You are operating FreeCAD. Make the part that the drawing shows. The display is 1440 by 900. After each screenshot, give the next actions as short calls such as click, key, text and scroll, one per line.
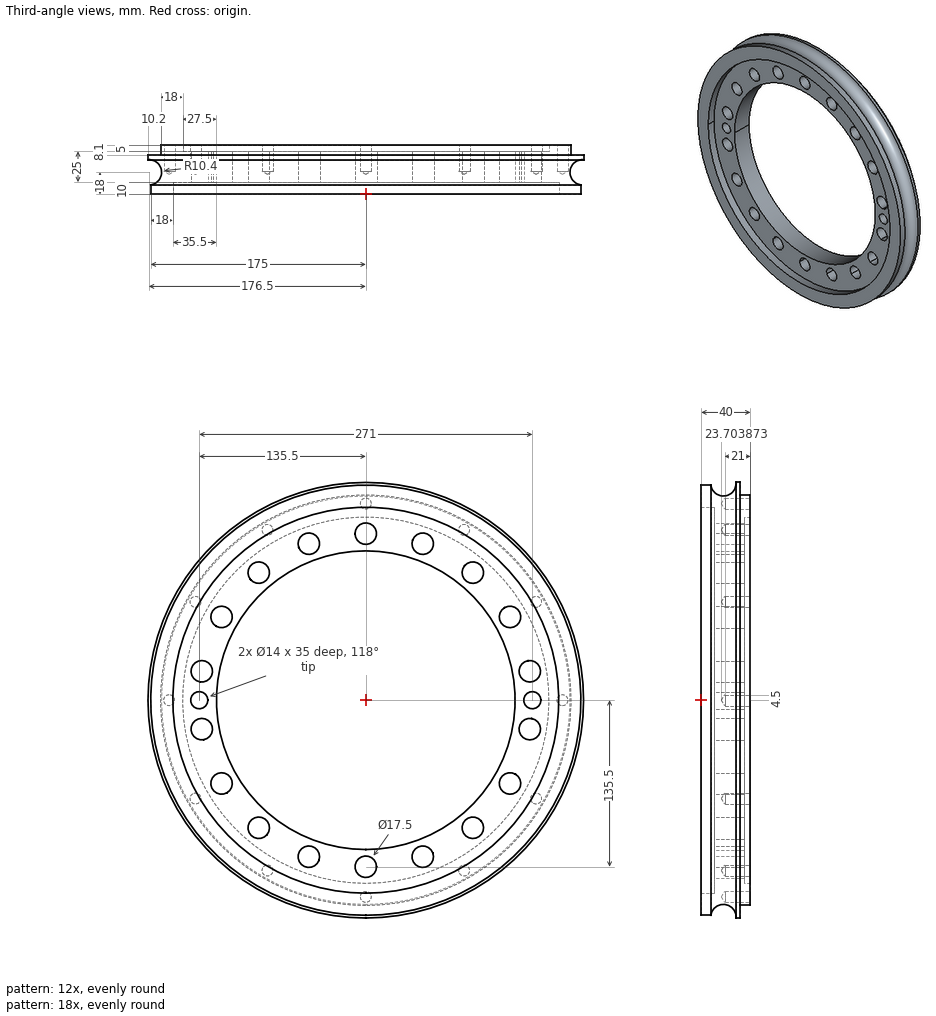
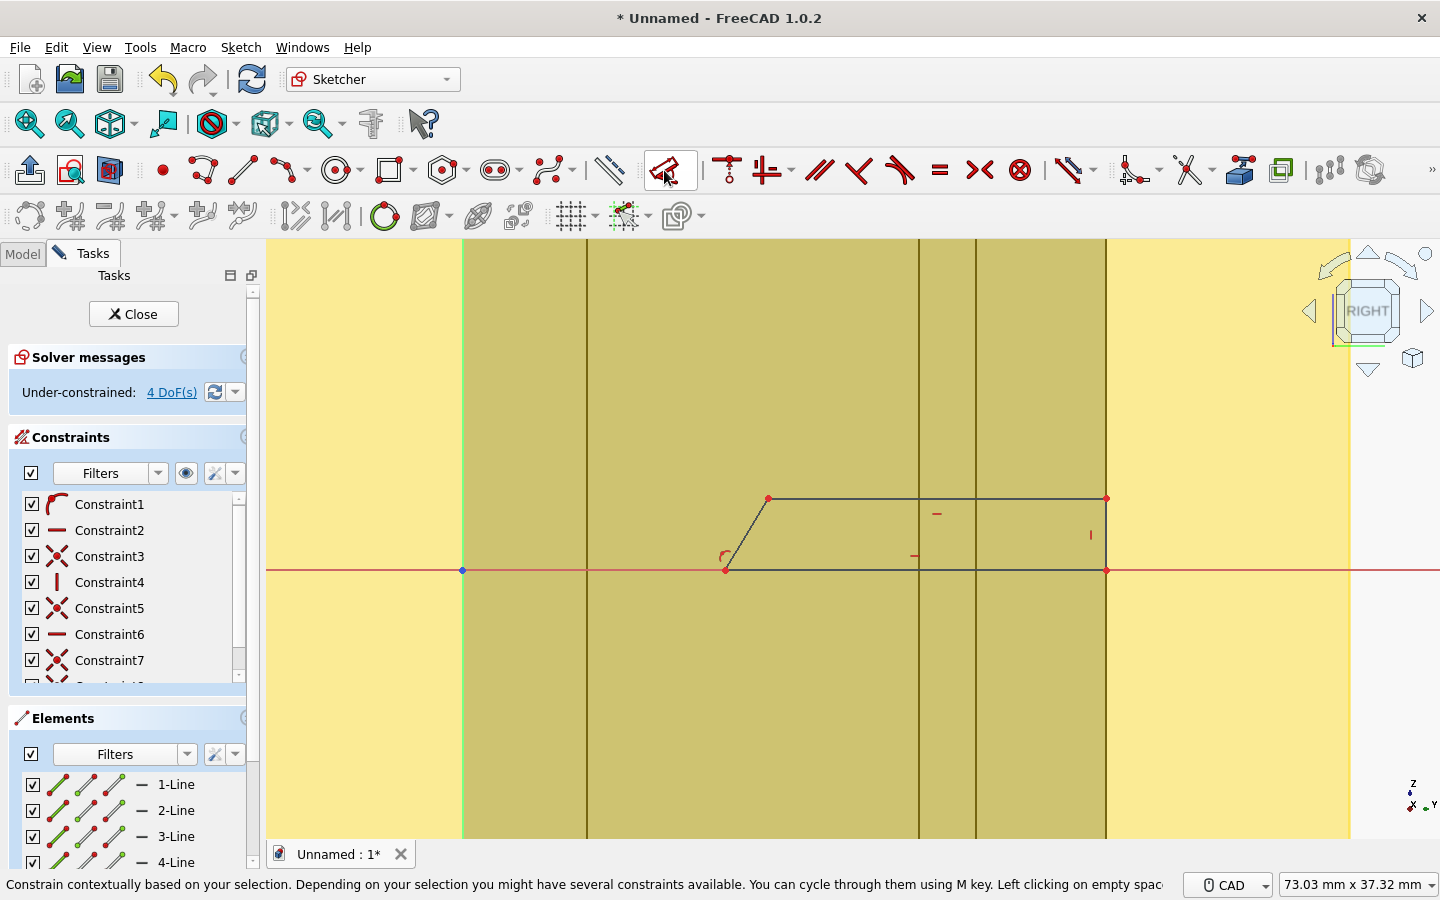
click(1005, 499)
click(937, 465)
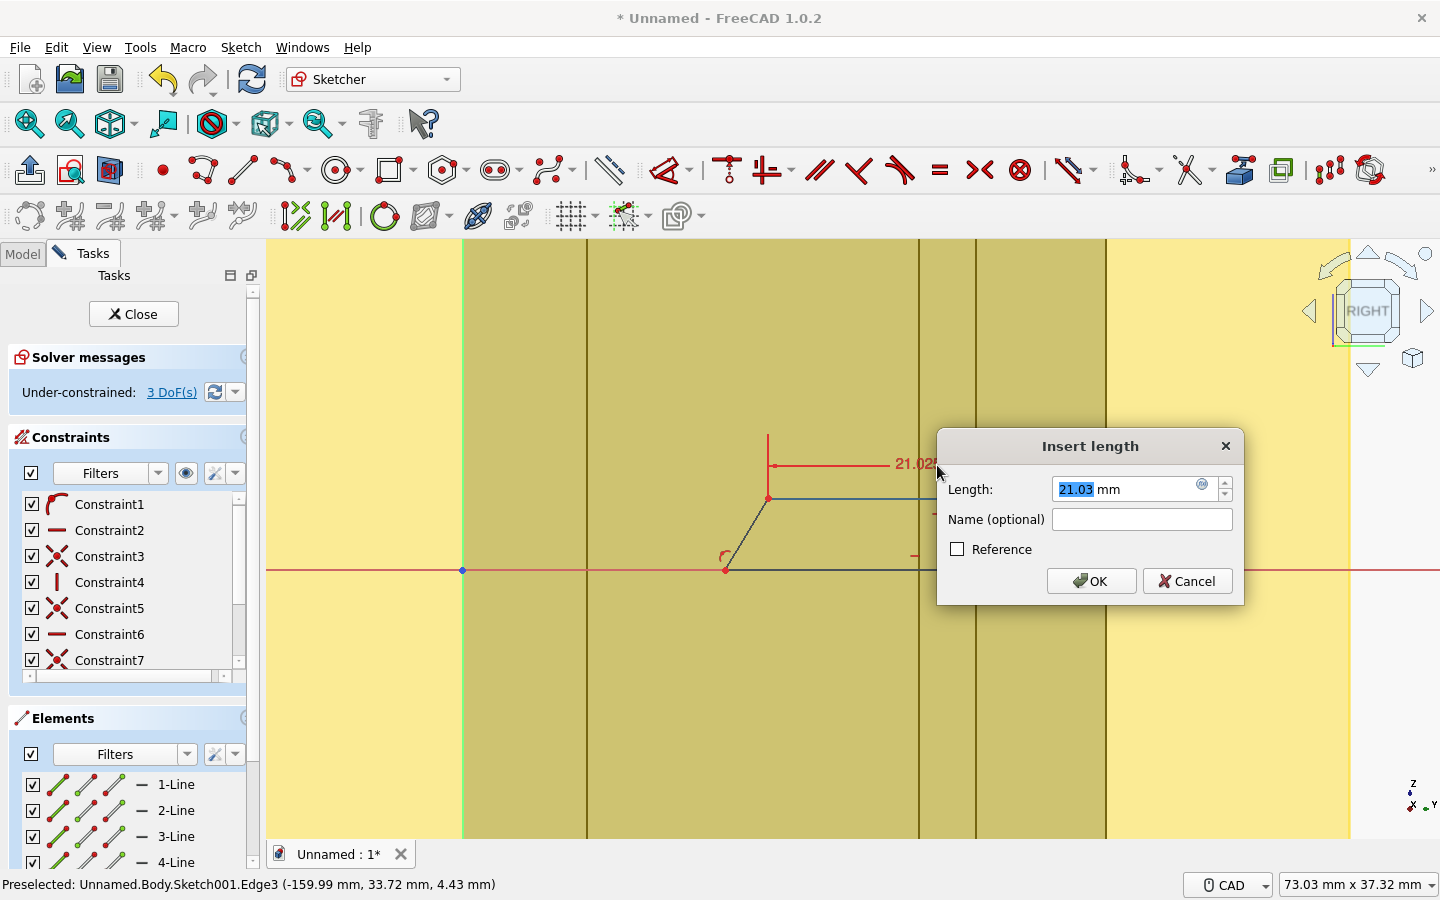
text(21)
key(Return)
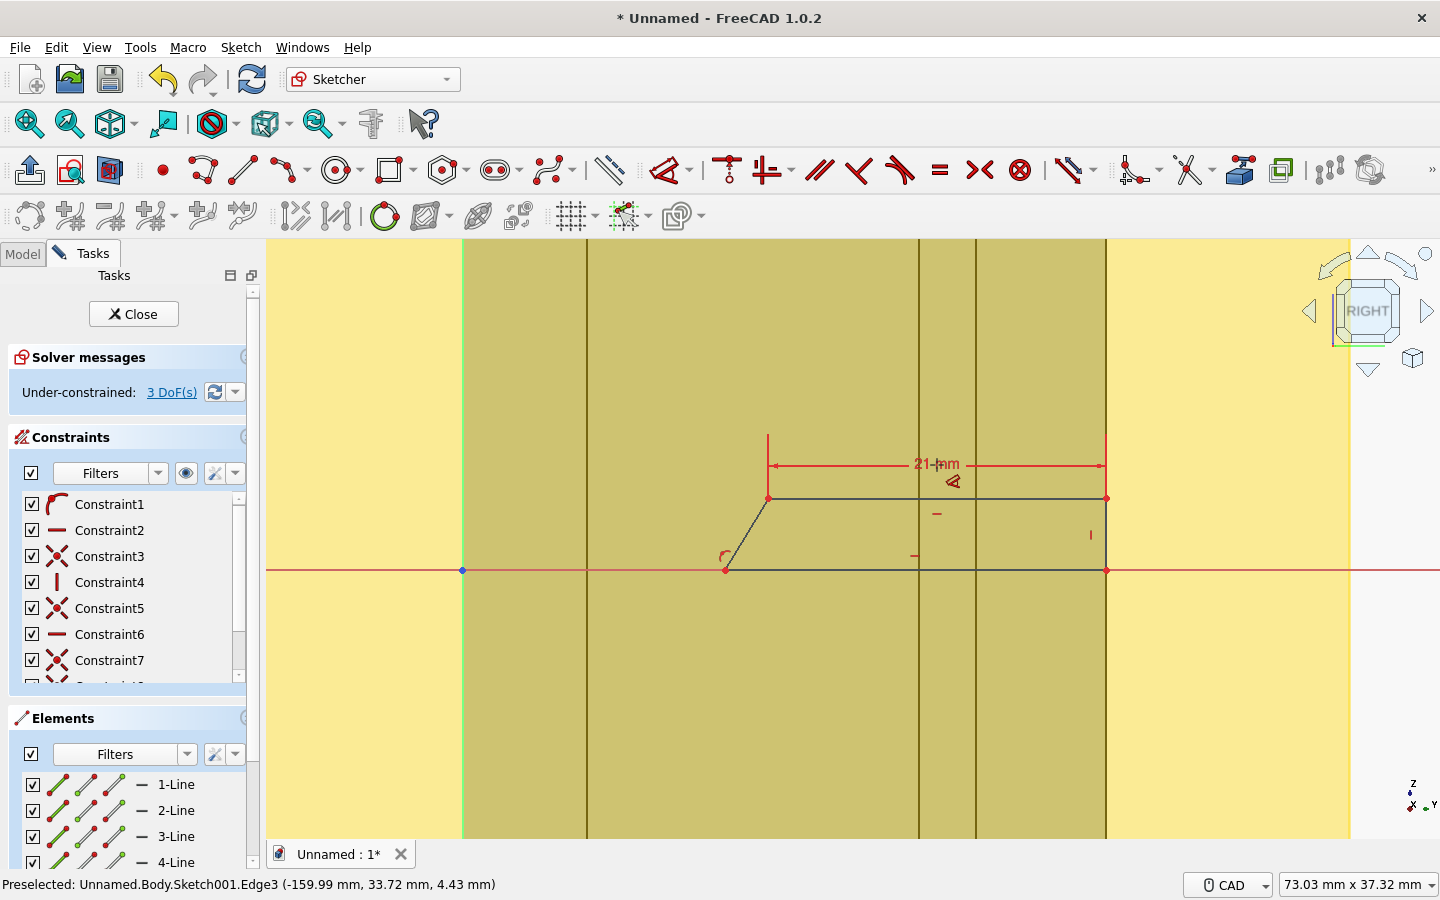
click(1106, 549)
click(1140, 535)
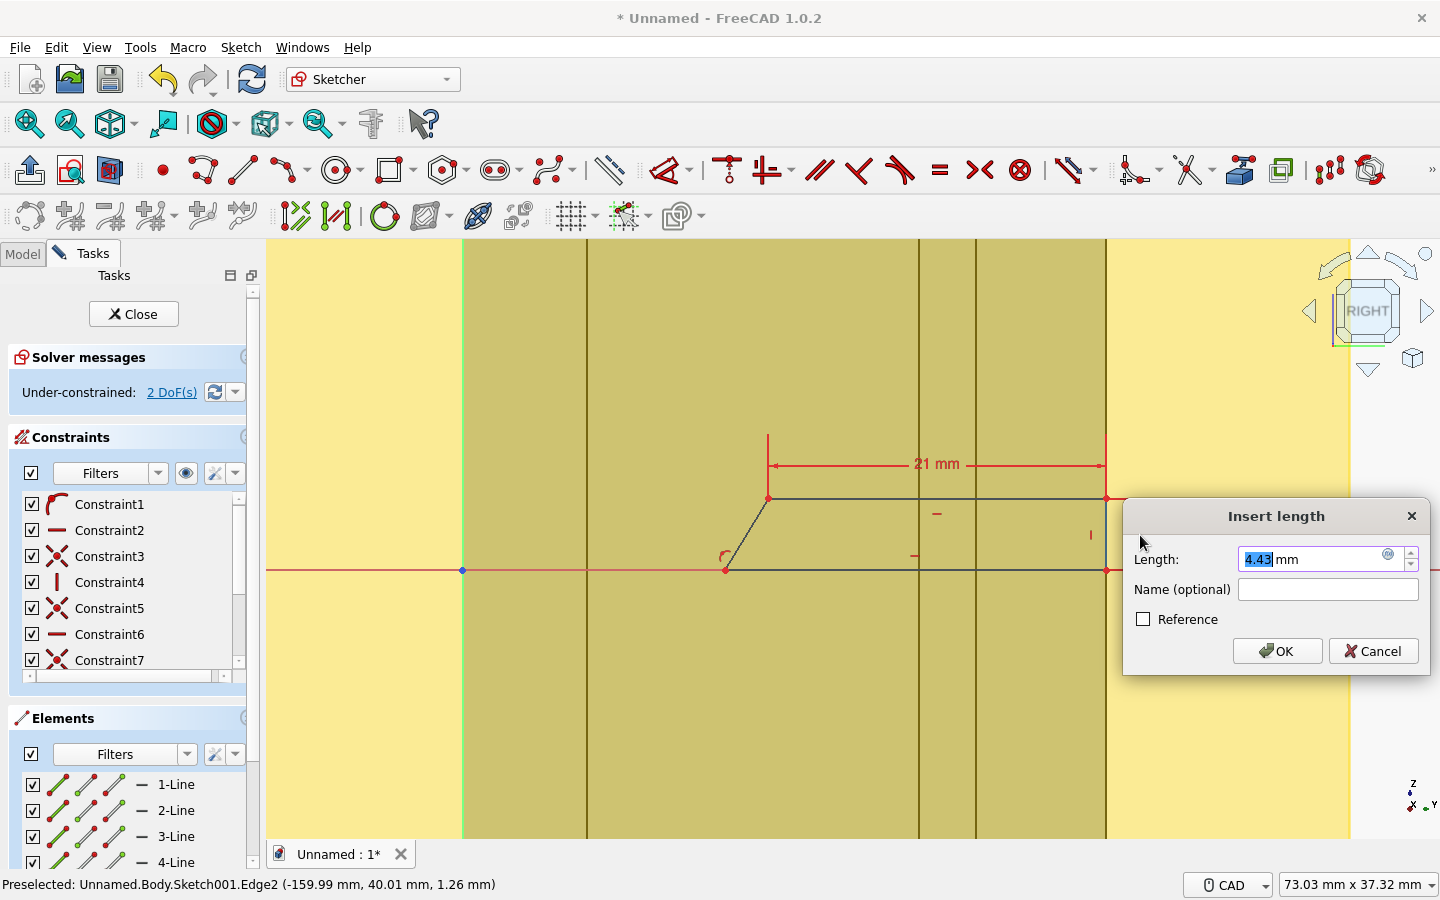
text(4.5)
key(Return)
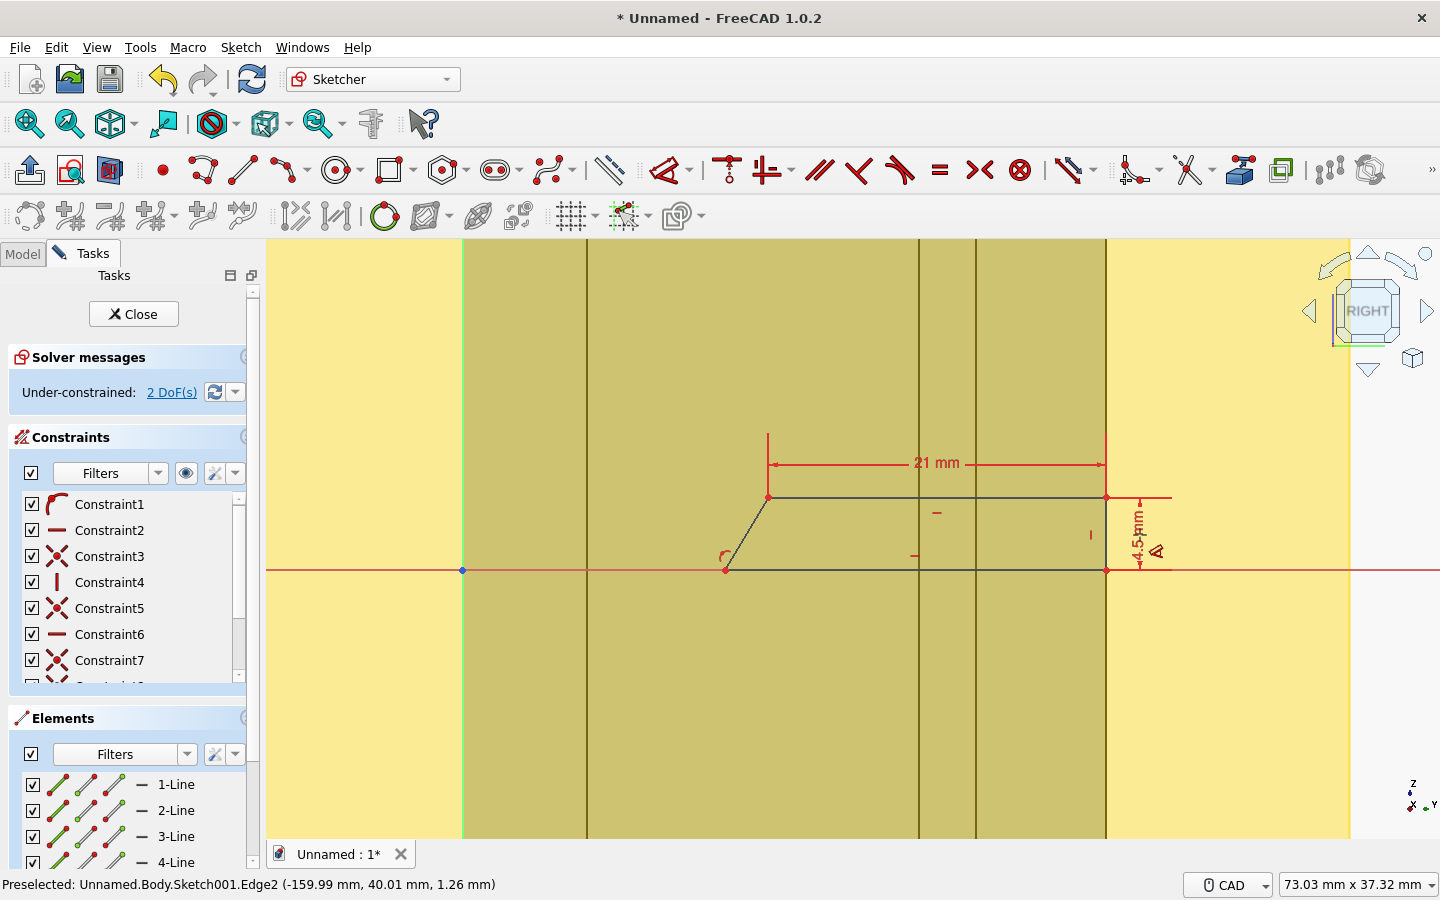
click(1106, 570)
click(784, 604)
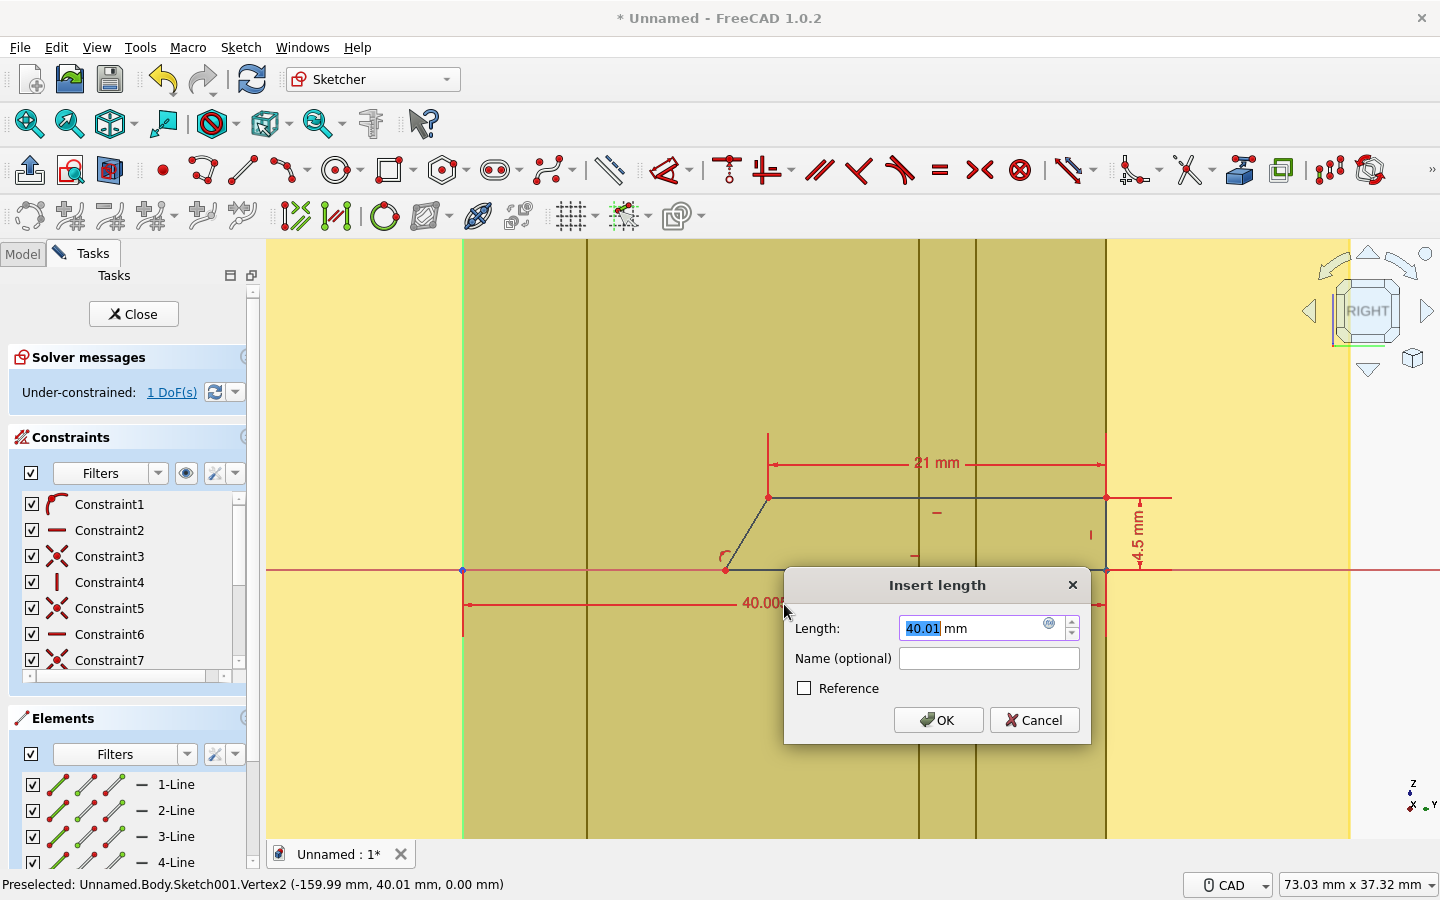
text(40)
key(Return)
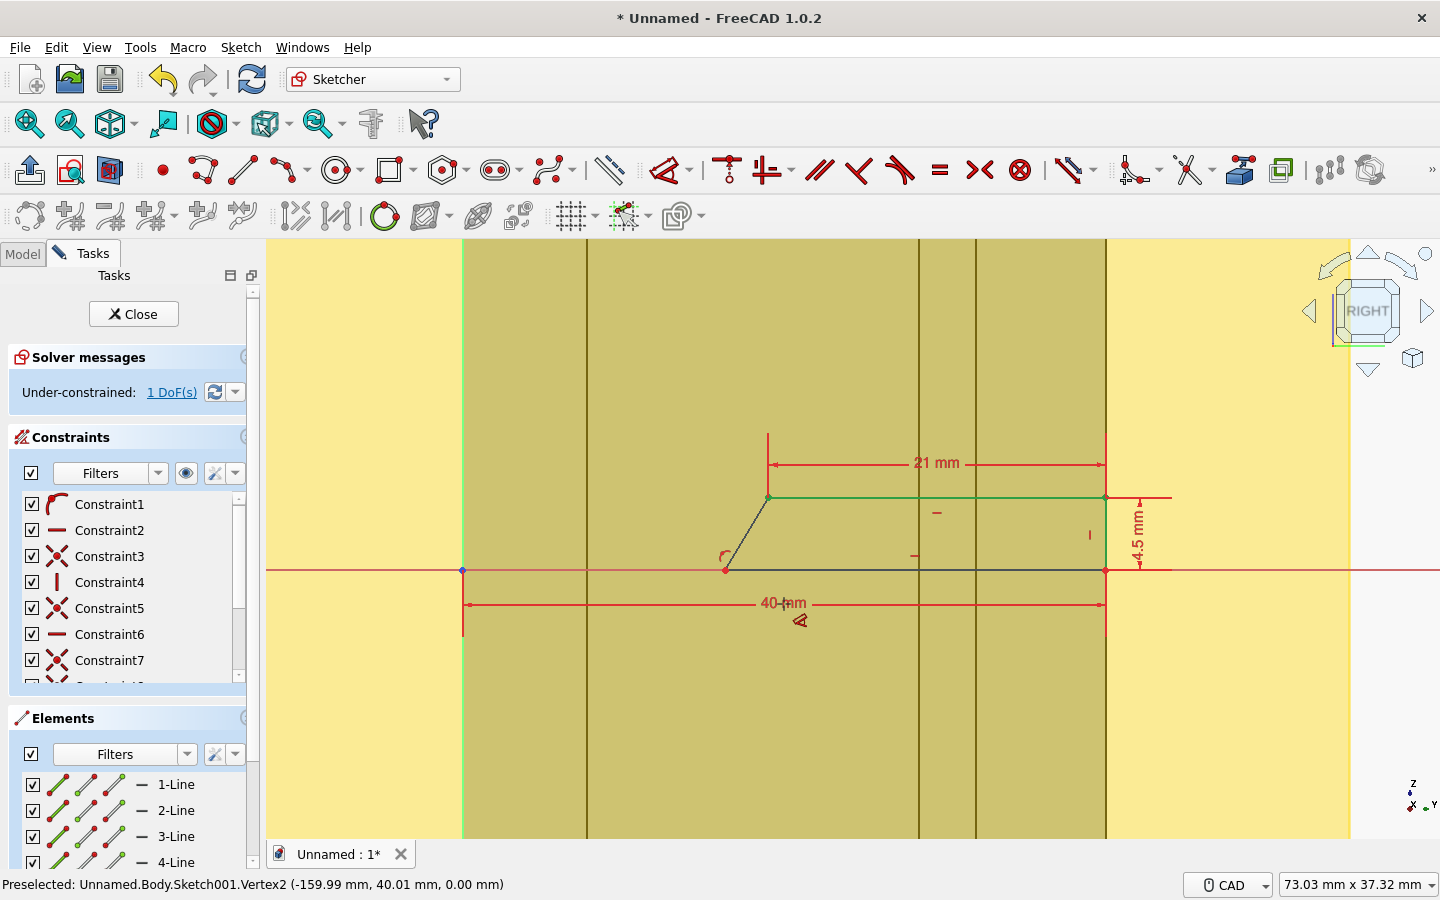
click(839, 570)
click(915, 604)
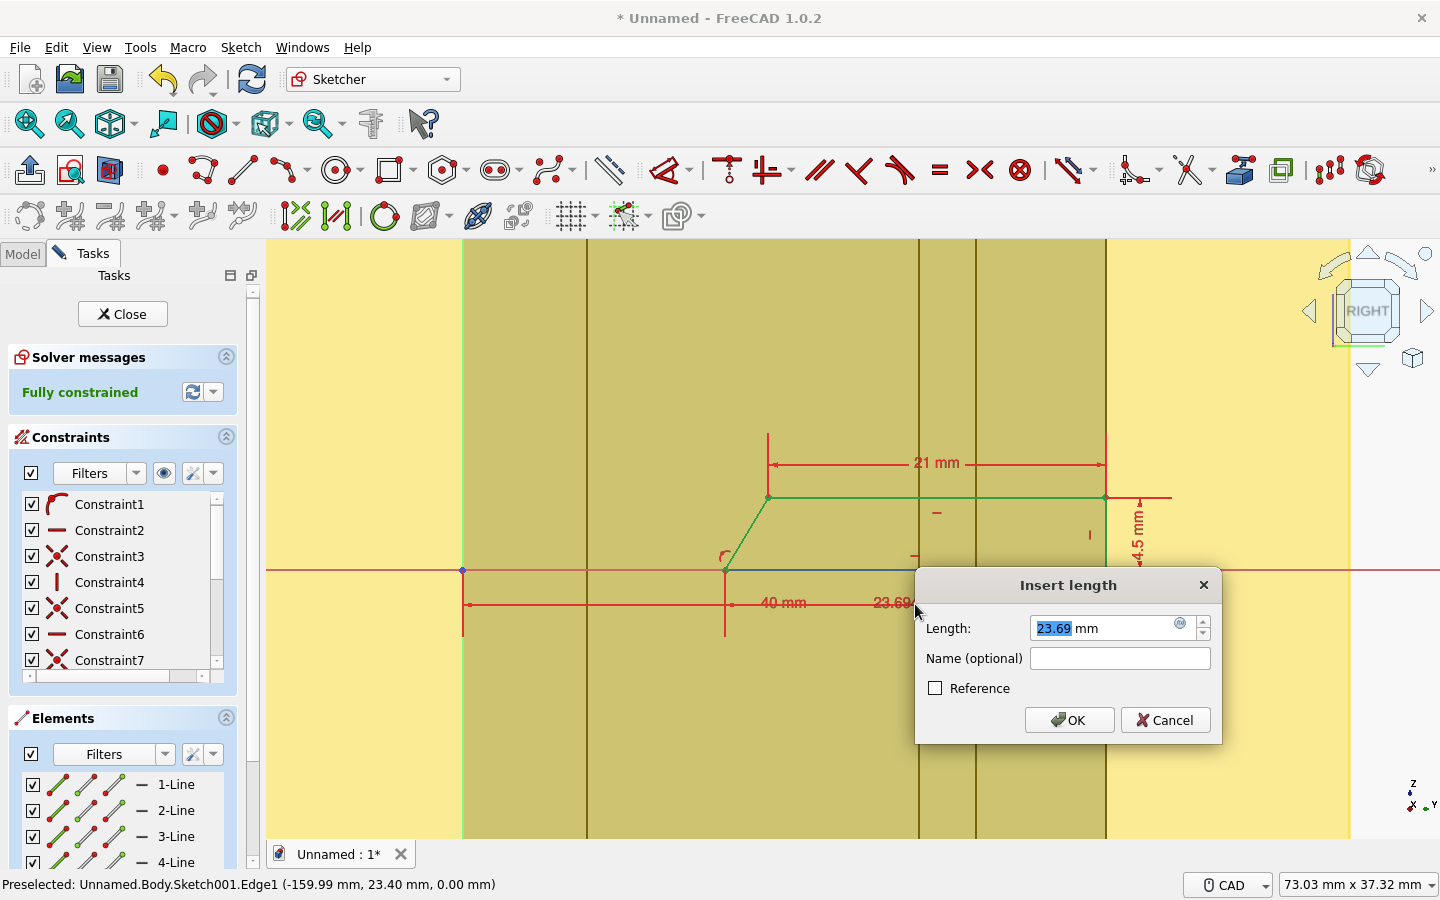
text(23.703873)
key(Return)
key(Escape)